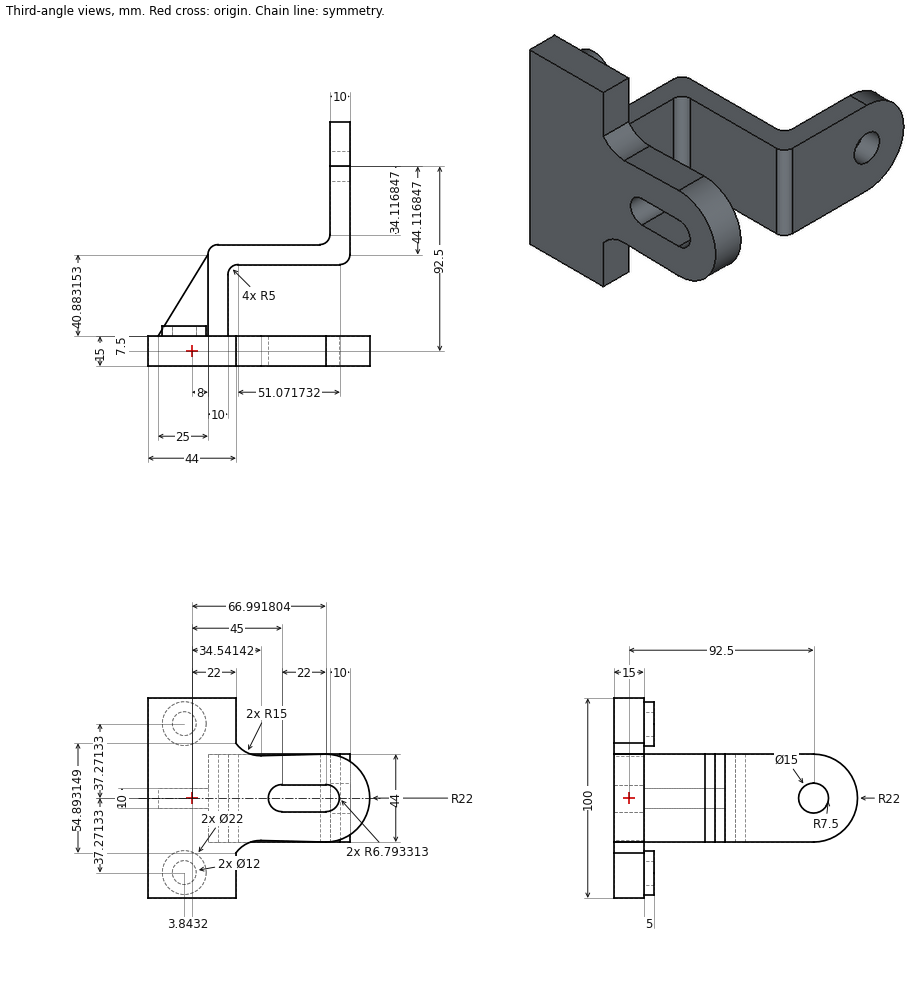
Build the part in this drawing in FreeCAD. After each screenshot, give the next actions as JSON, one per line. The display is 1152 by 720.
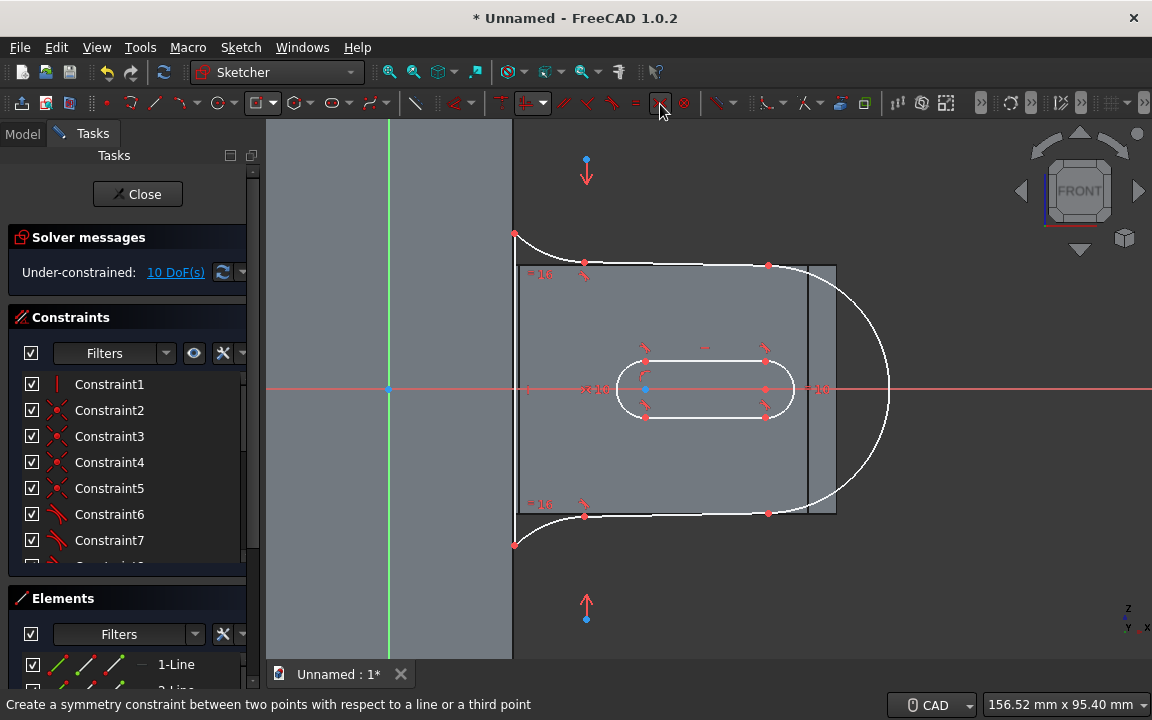
{"action": "left_click", "coordinate": [454, 104]}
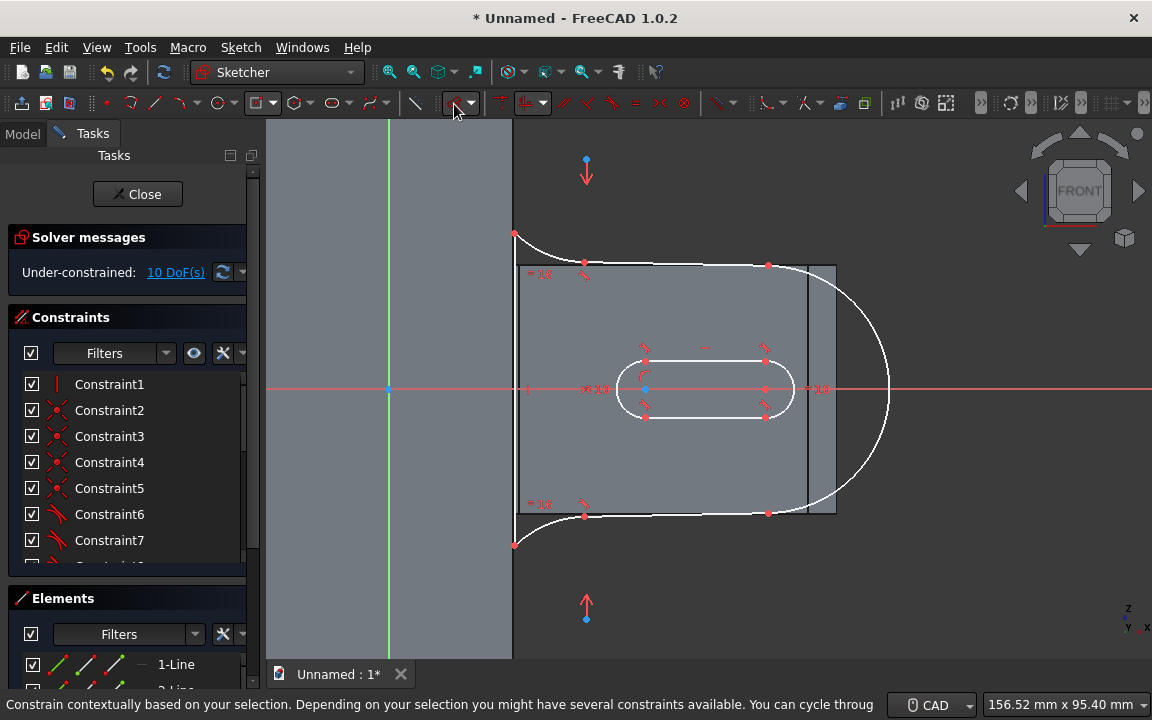
{"action": "left_click", "coordinate": [533, 247]}
{"action": "left_click", "coordinate": [470, 227]}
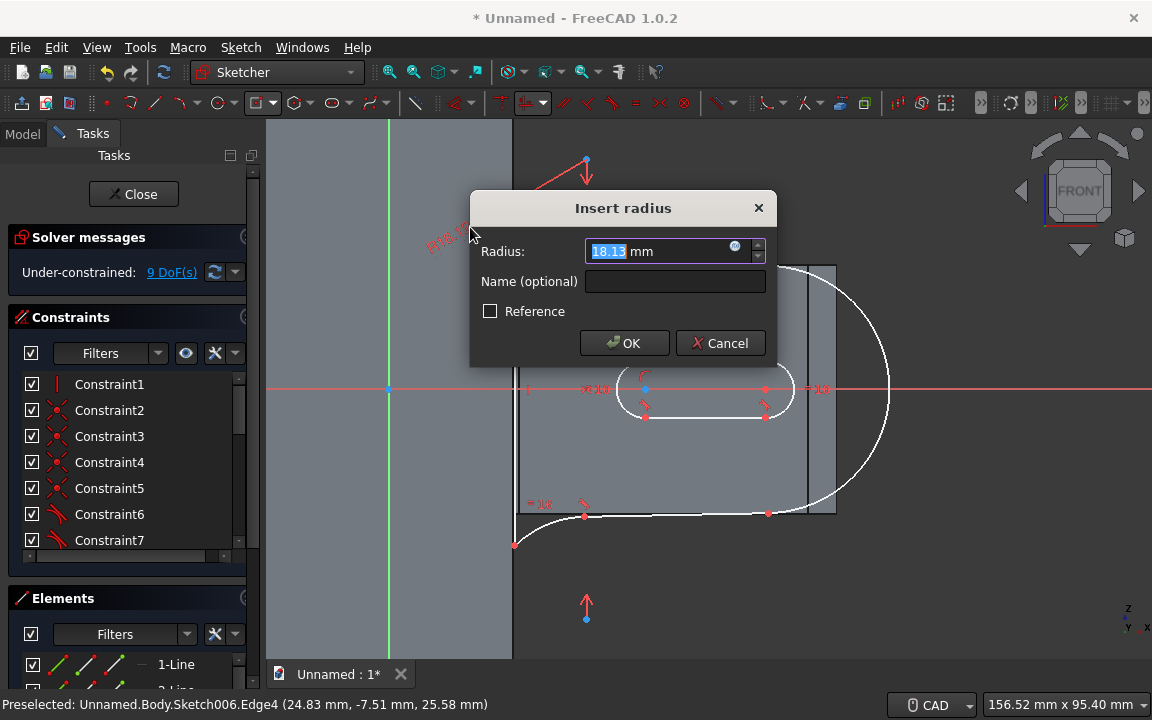
{"action": "type", "text": "15"}
{"action": "key", "text": "Return"}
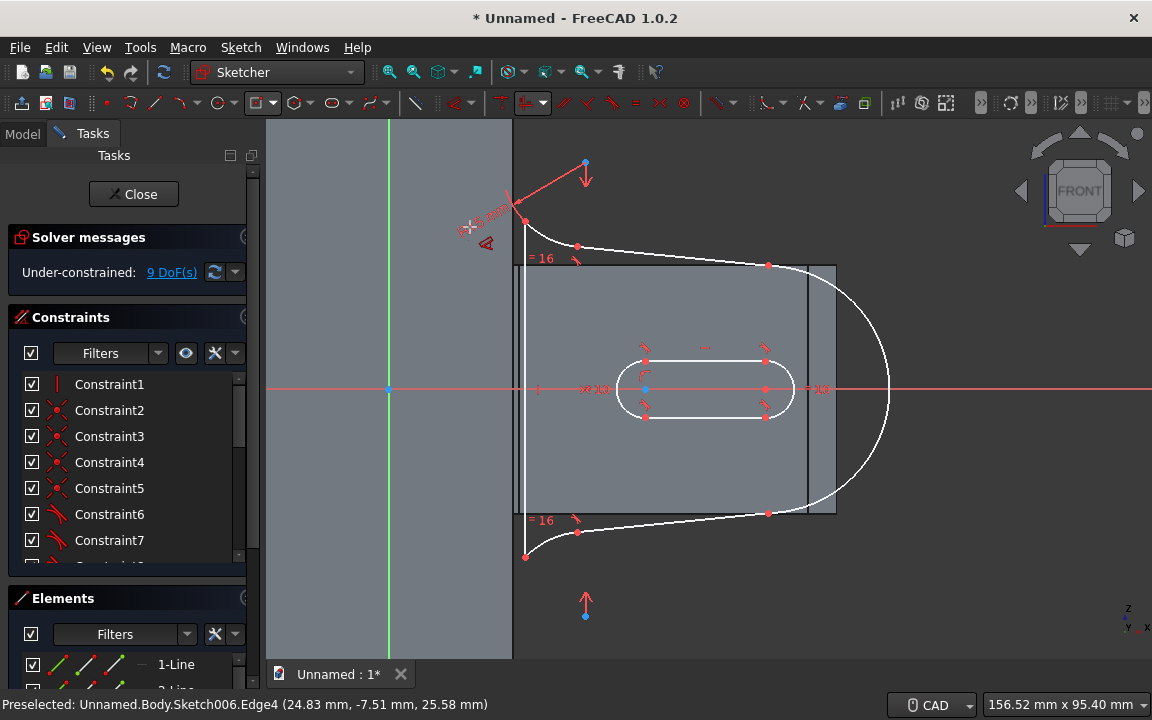
{"action": "left_click", "coordinate": [866, 461]}
{"action": "left_click", "coordinate": [892, 480]}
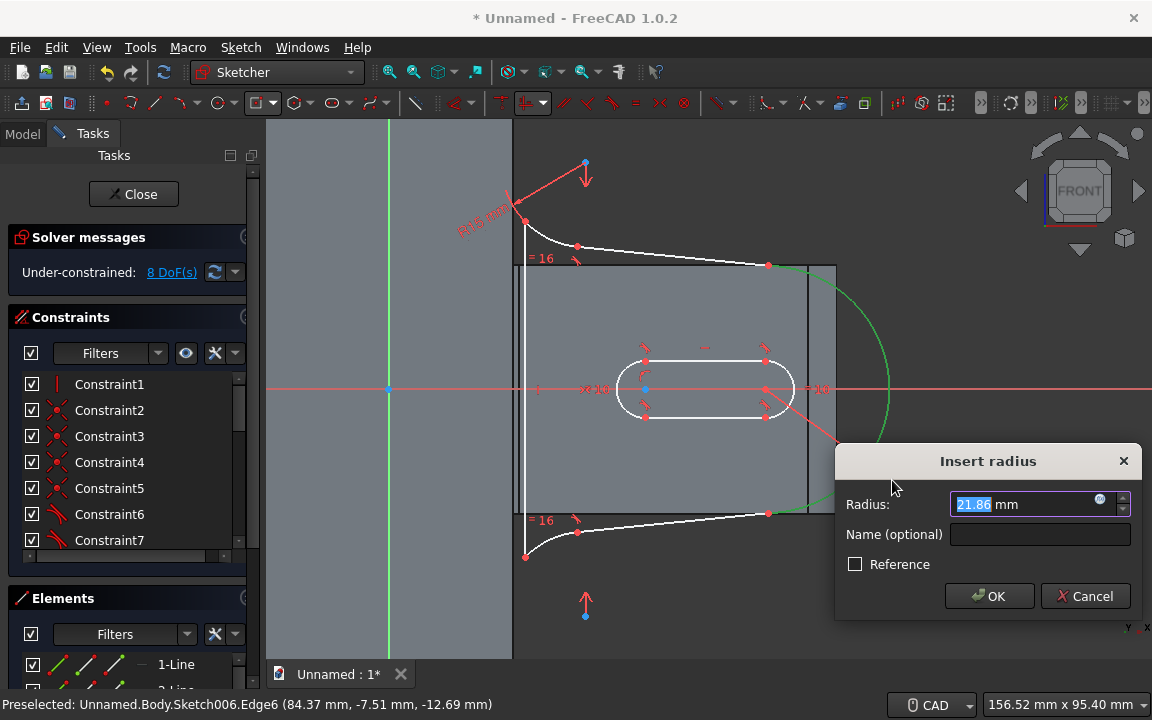
{"action": "type", "text": "22"}
{"action": "key", "text": "Return"}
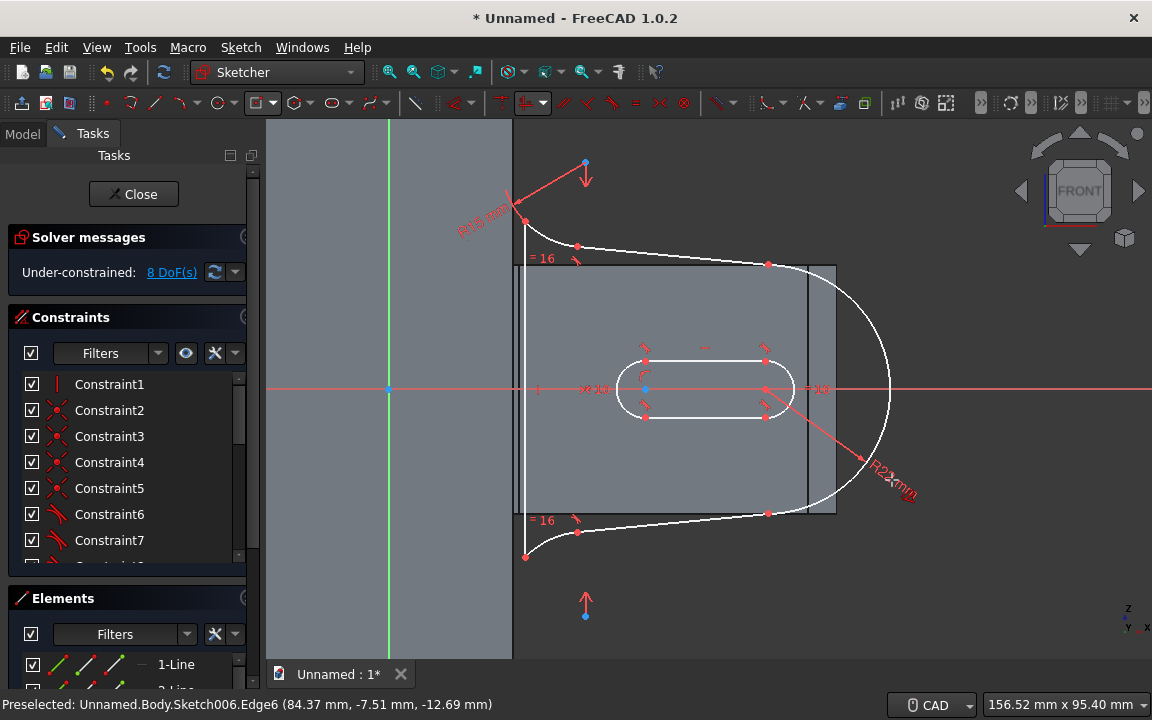
{"action": "left_click", "coordinate": [622, 373]}
{"action": "left_click", "coordinate": [596, 355]}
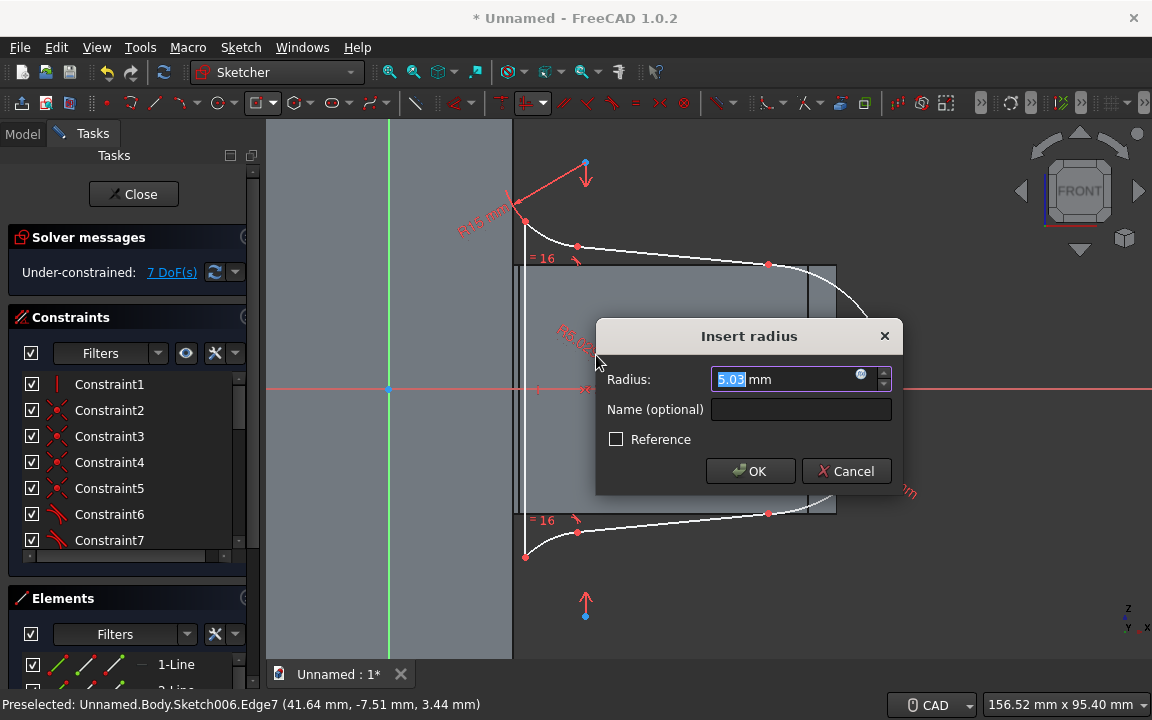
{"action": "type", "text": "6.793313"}
{"action": "key", "text": "Return"}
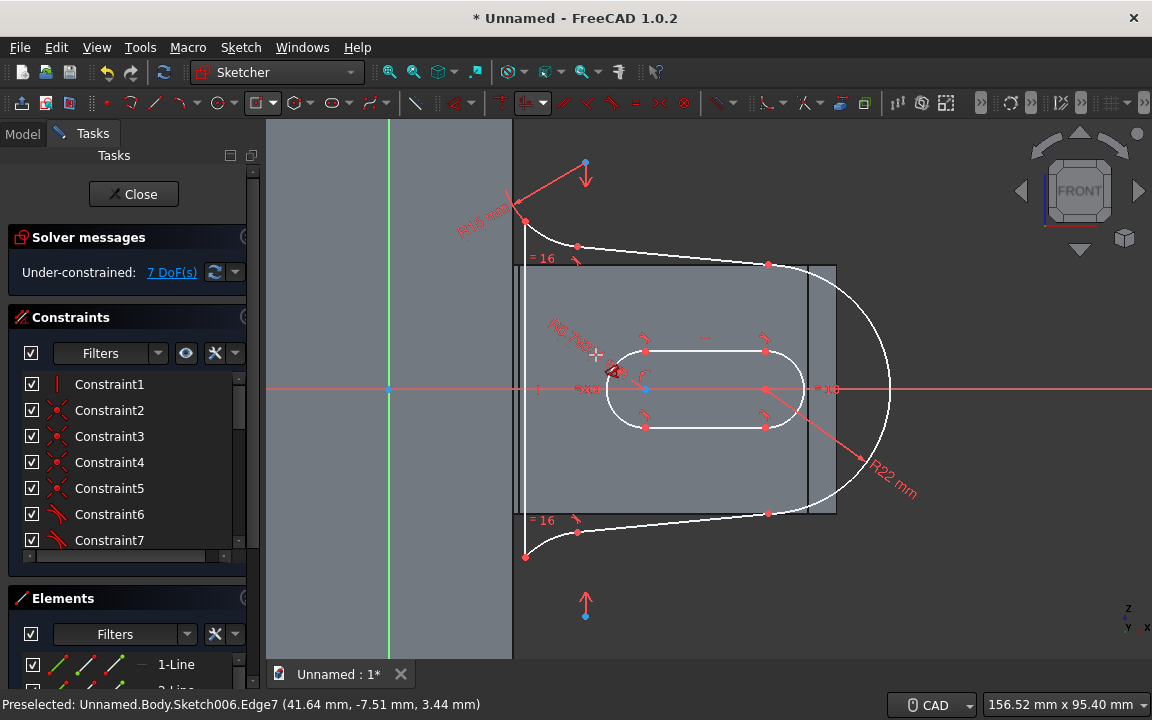
{"action": "left_click", "coordinate": [681, 351]}
{"action": "left_click", "coordinate": [705, 317]}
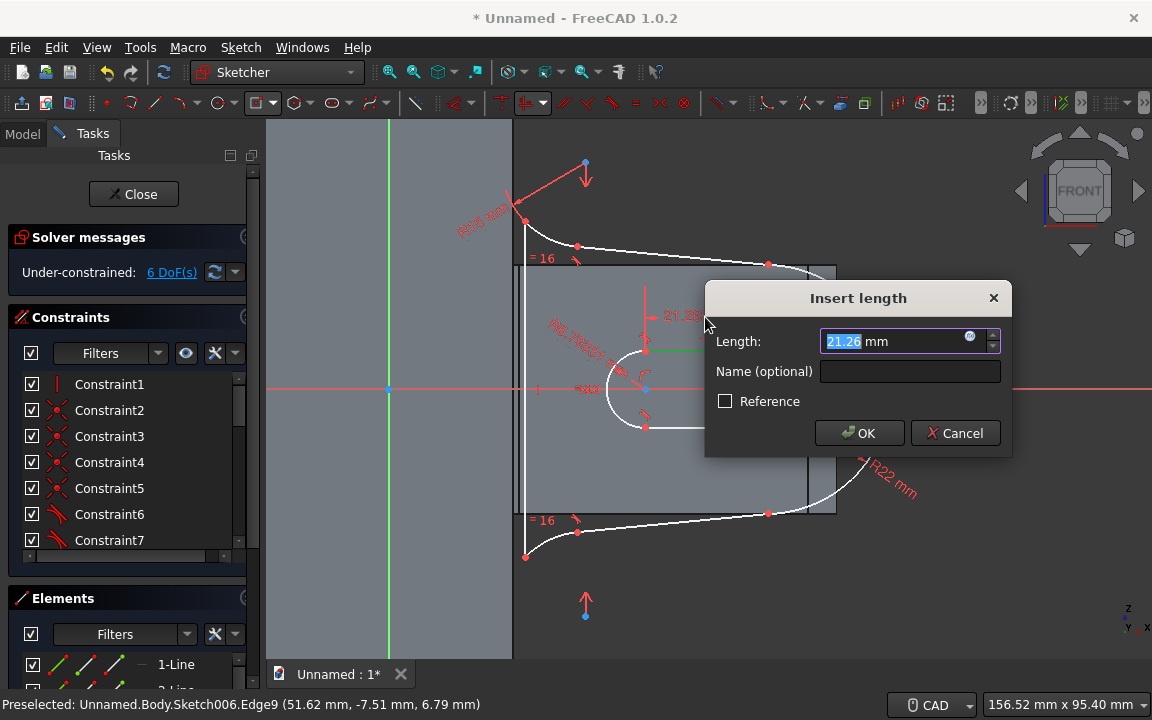
{"action": "type", "text": "22"}
{"action": "key", "text": "Return"}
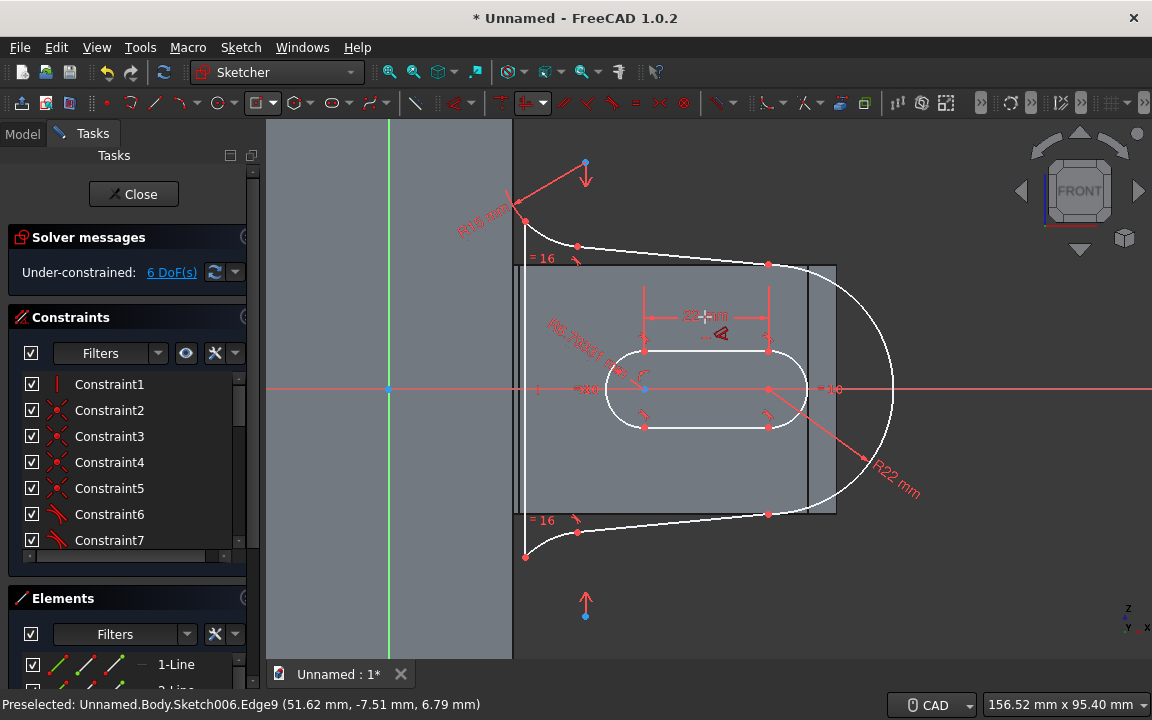
{"action": "left_click", "coordinate": [525, 222]}
{"action": "left_click", "coordinate": [457, 188]}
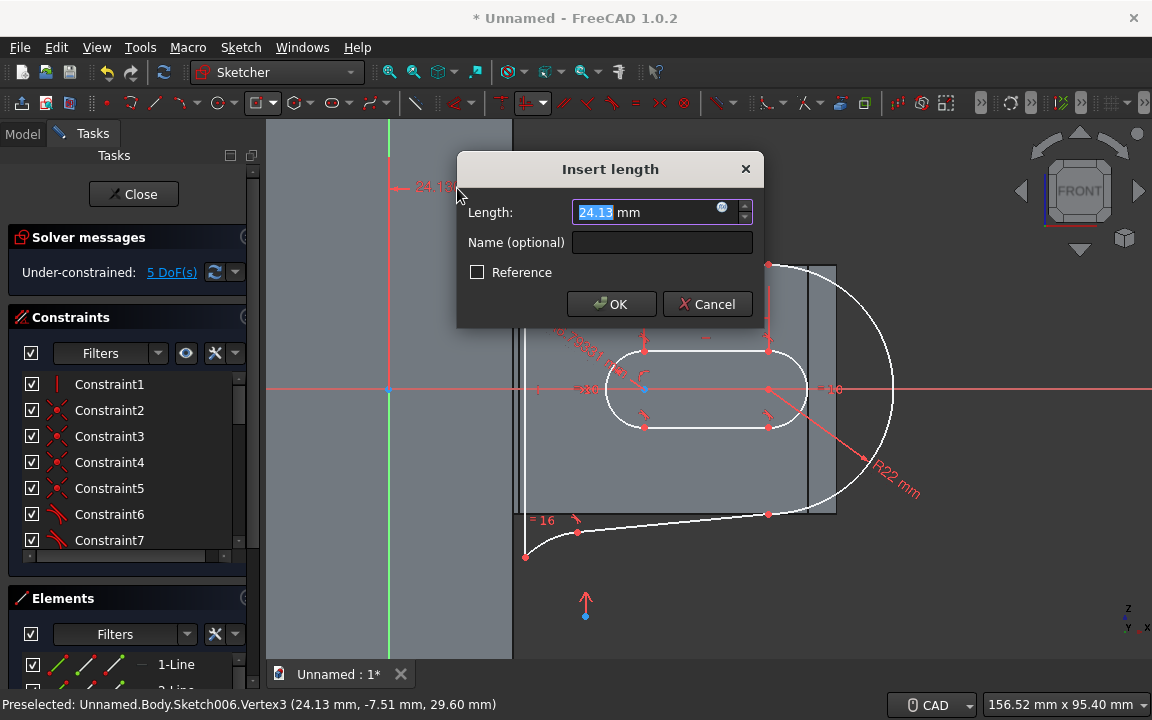
{"action": "type", "text": "22"}
{"action": "key", "text": "Return"}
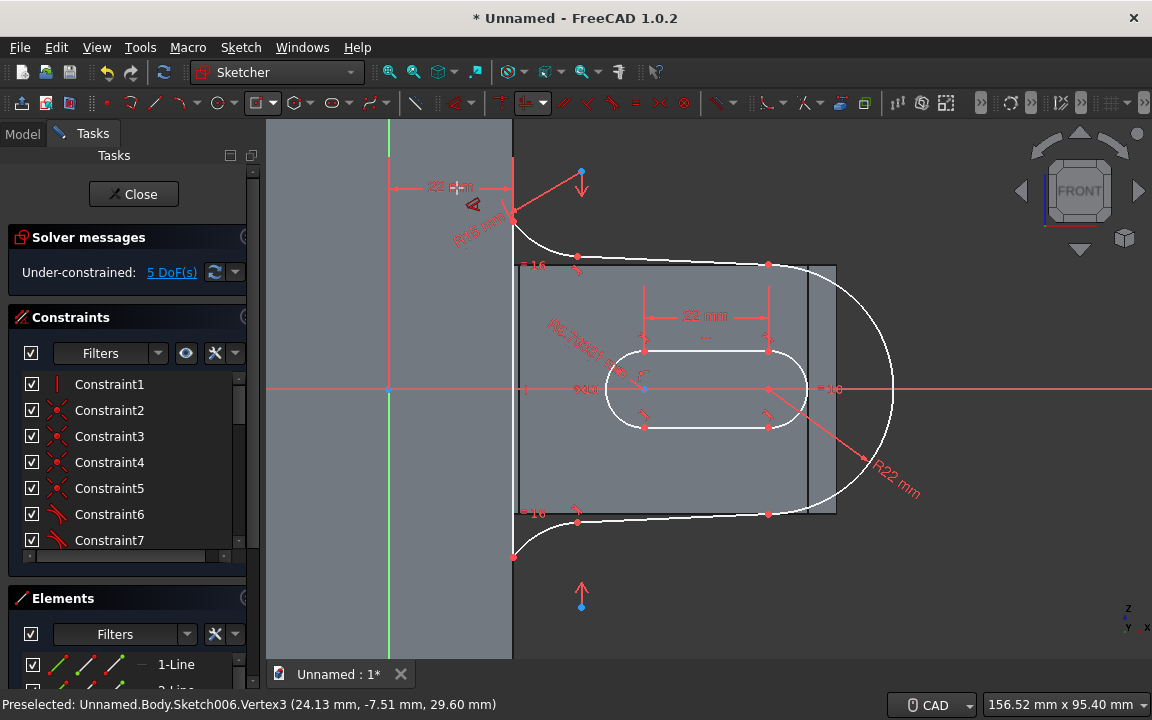
{"action": "left_click", "coordinate": [644, 351]}
{"action": "left_click", "coordinate": [458, 317]}